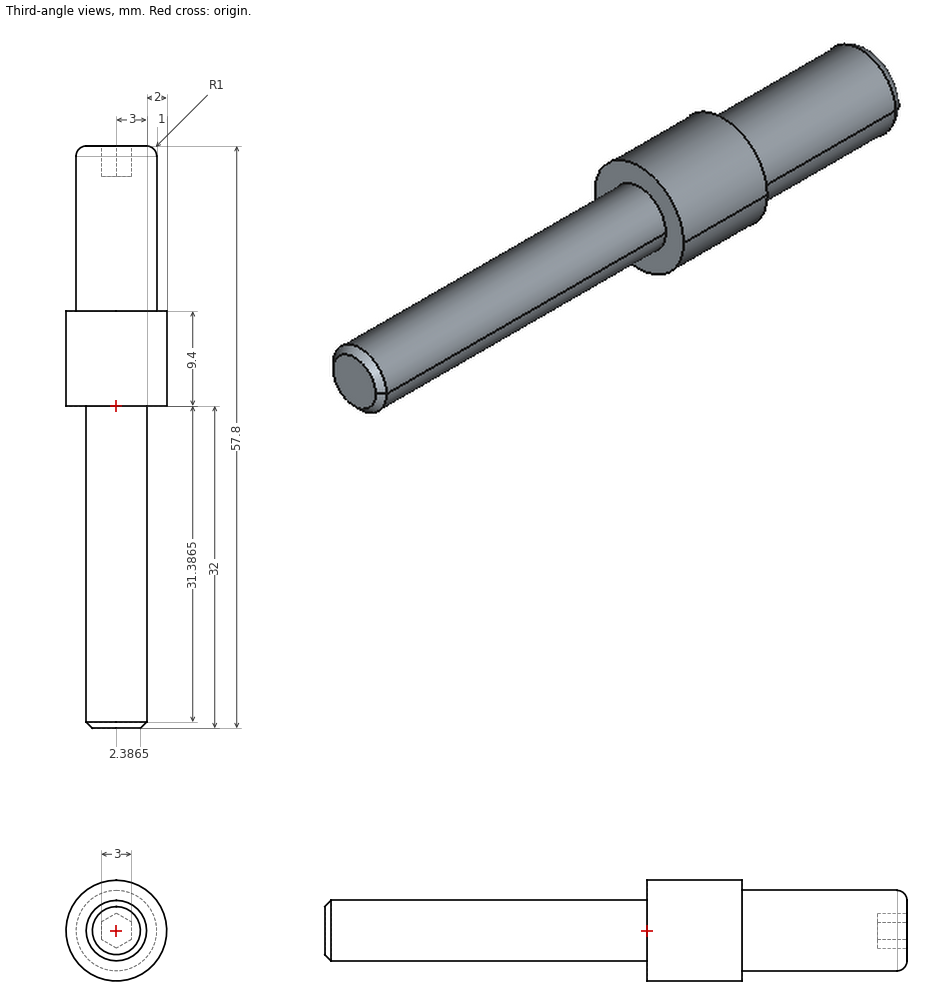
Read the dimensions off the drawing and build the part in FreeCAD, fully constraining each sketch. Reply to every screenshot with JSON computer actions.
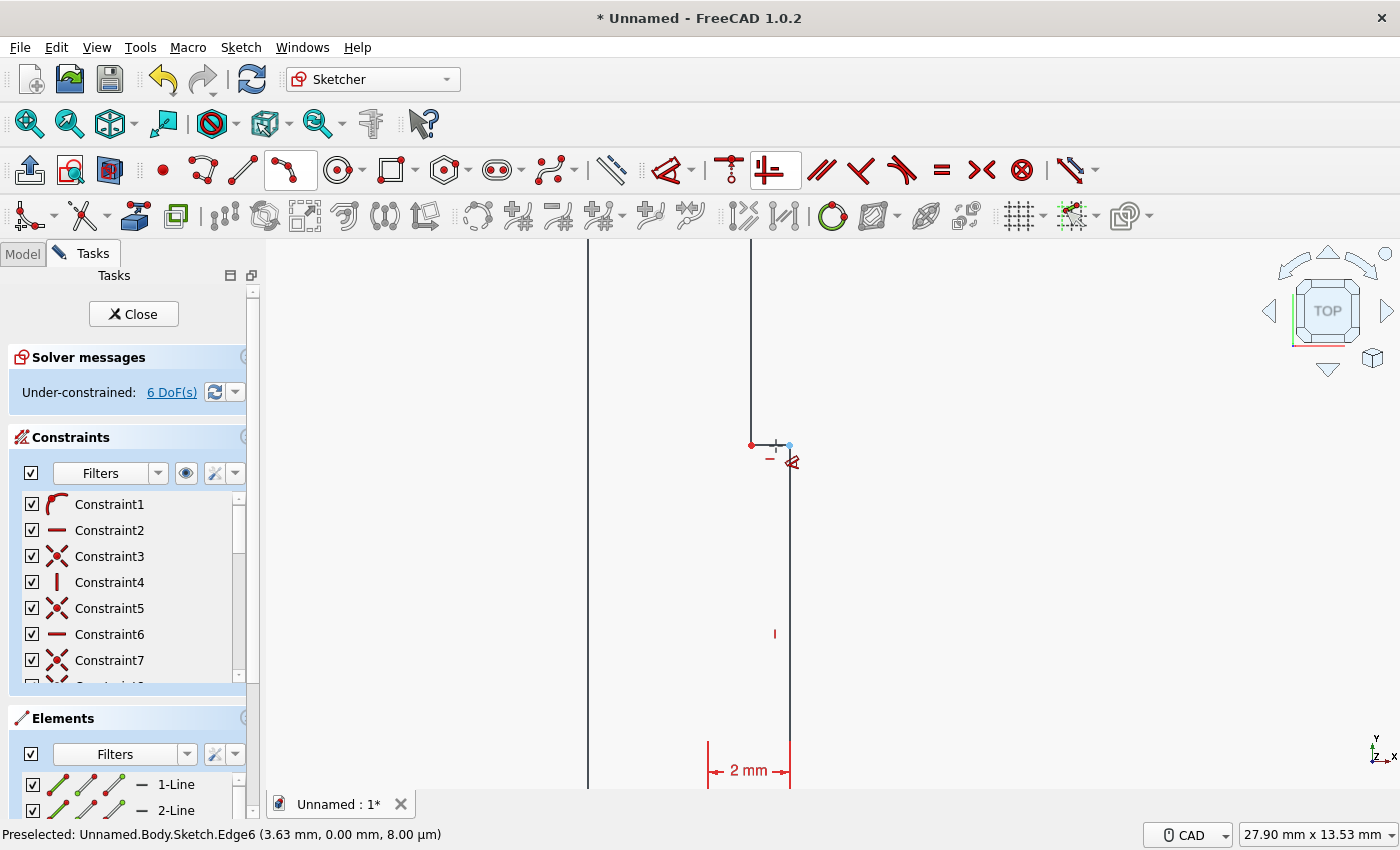
{"action": "left_click", "coordinate": [774, 445]}
{"action": "left_click", "coordinate": [770, 411]}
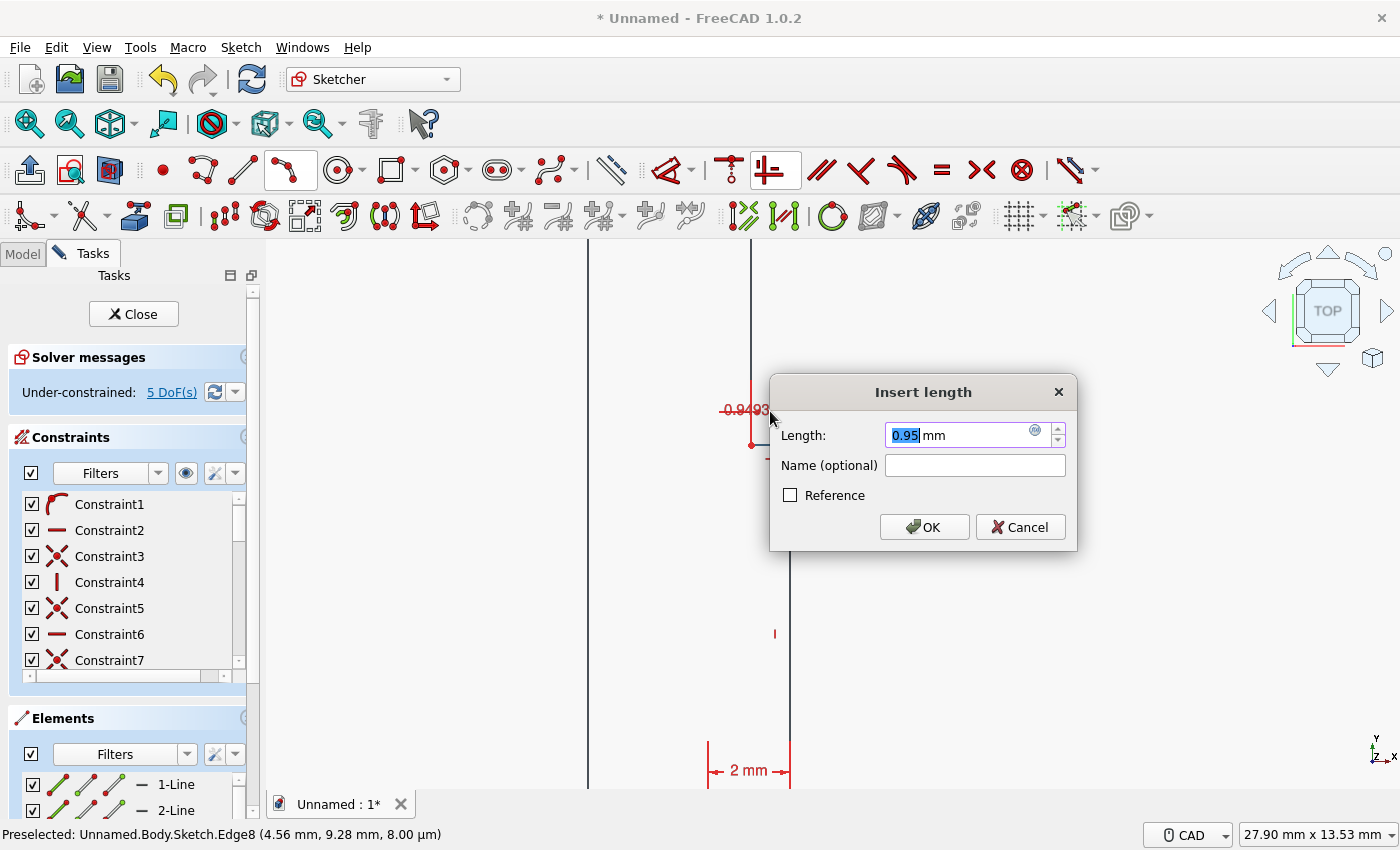
{"action": "type", "text": "1"}
{"action": "key", "text": "Return"}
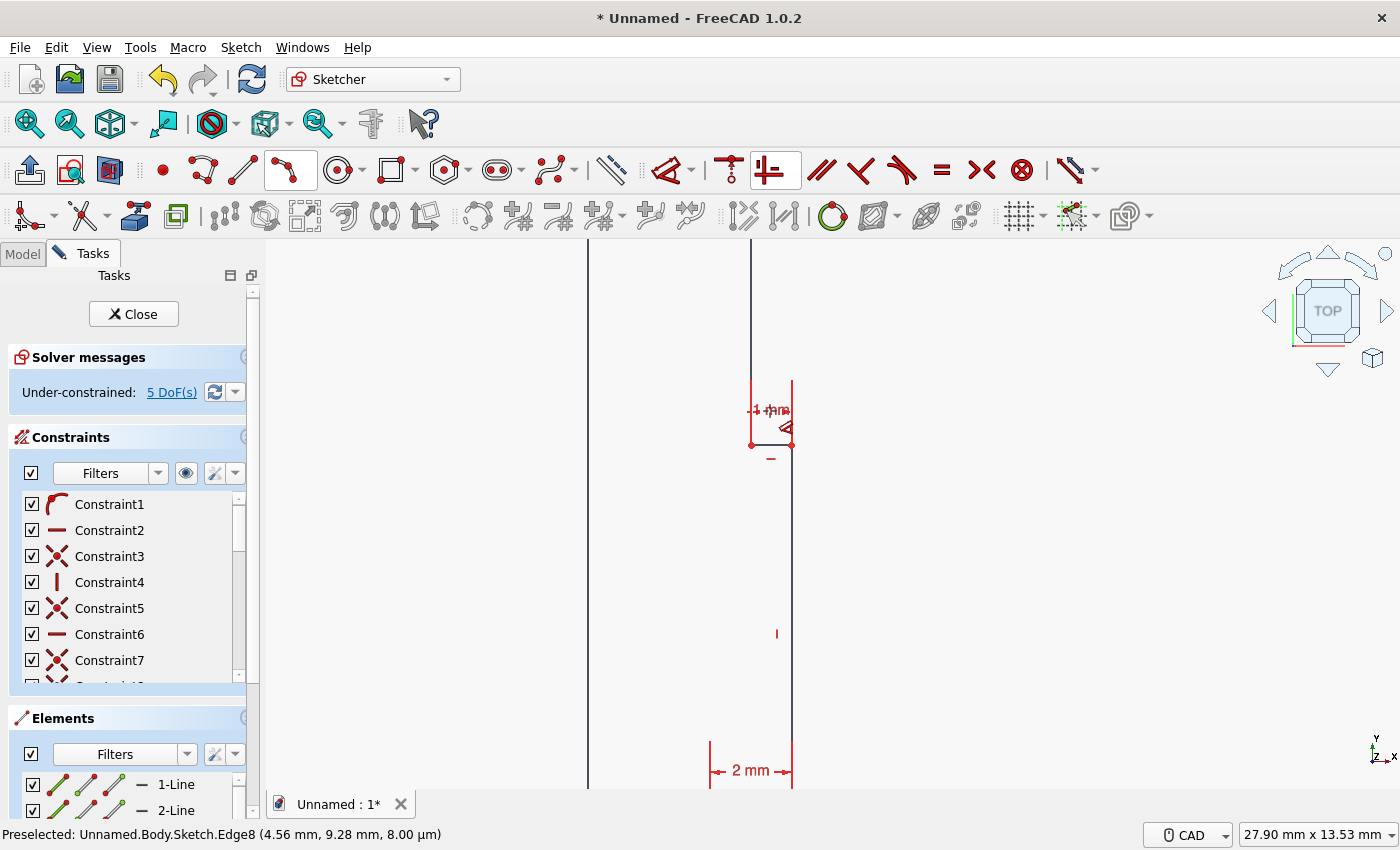
{"action": "scroll", "coordinate": [776, 446], "scroll_direction": "down", "scroll_amount": 10}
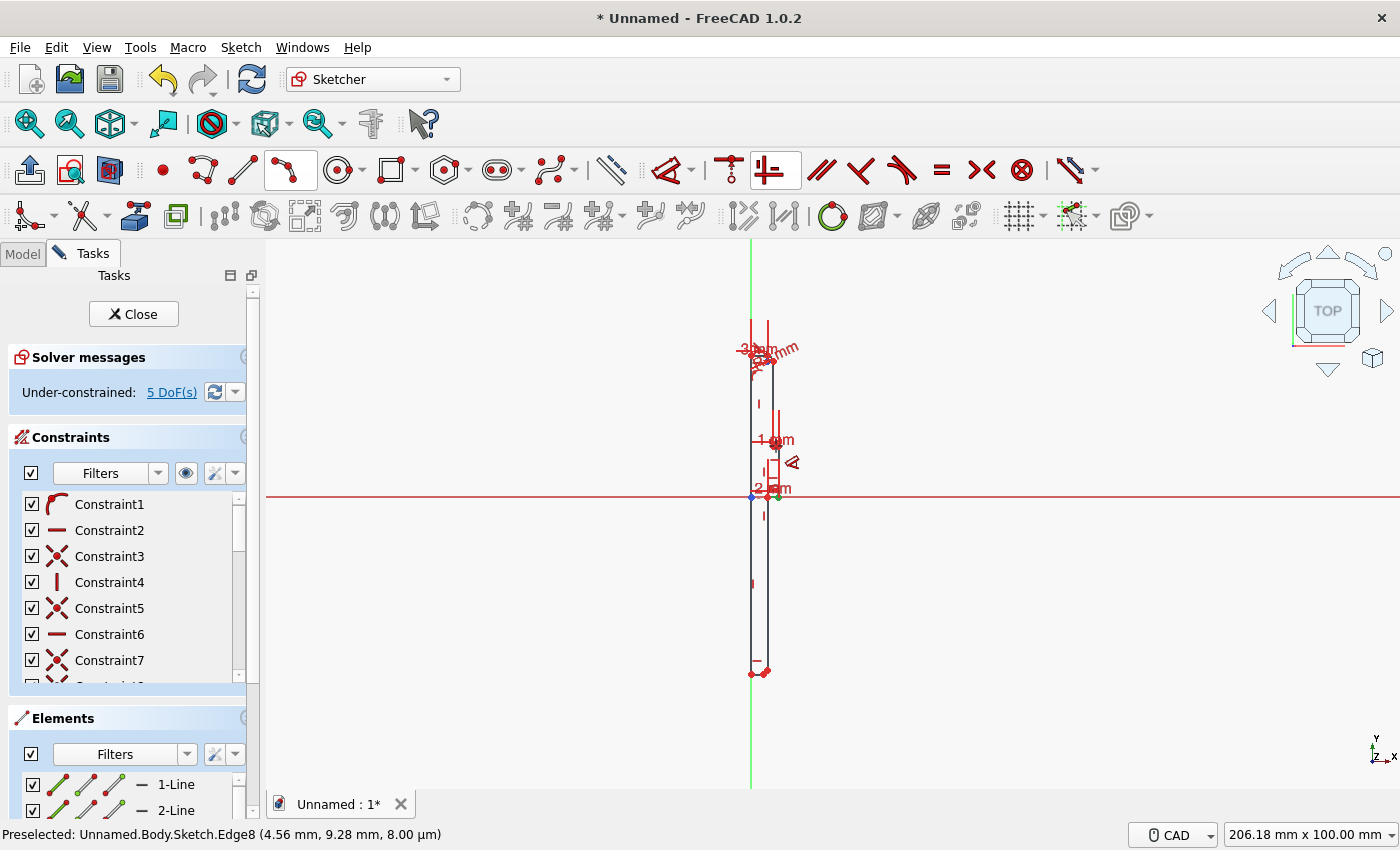
{"action": "left_click", "coordinate": [779, 482]}
{"action": "left_click", "coordinate": [861, 472]}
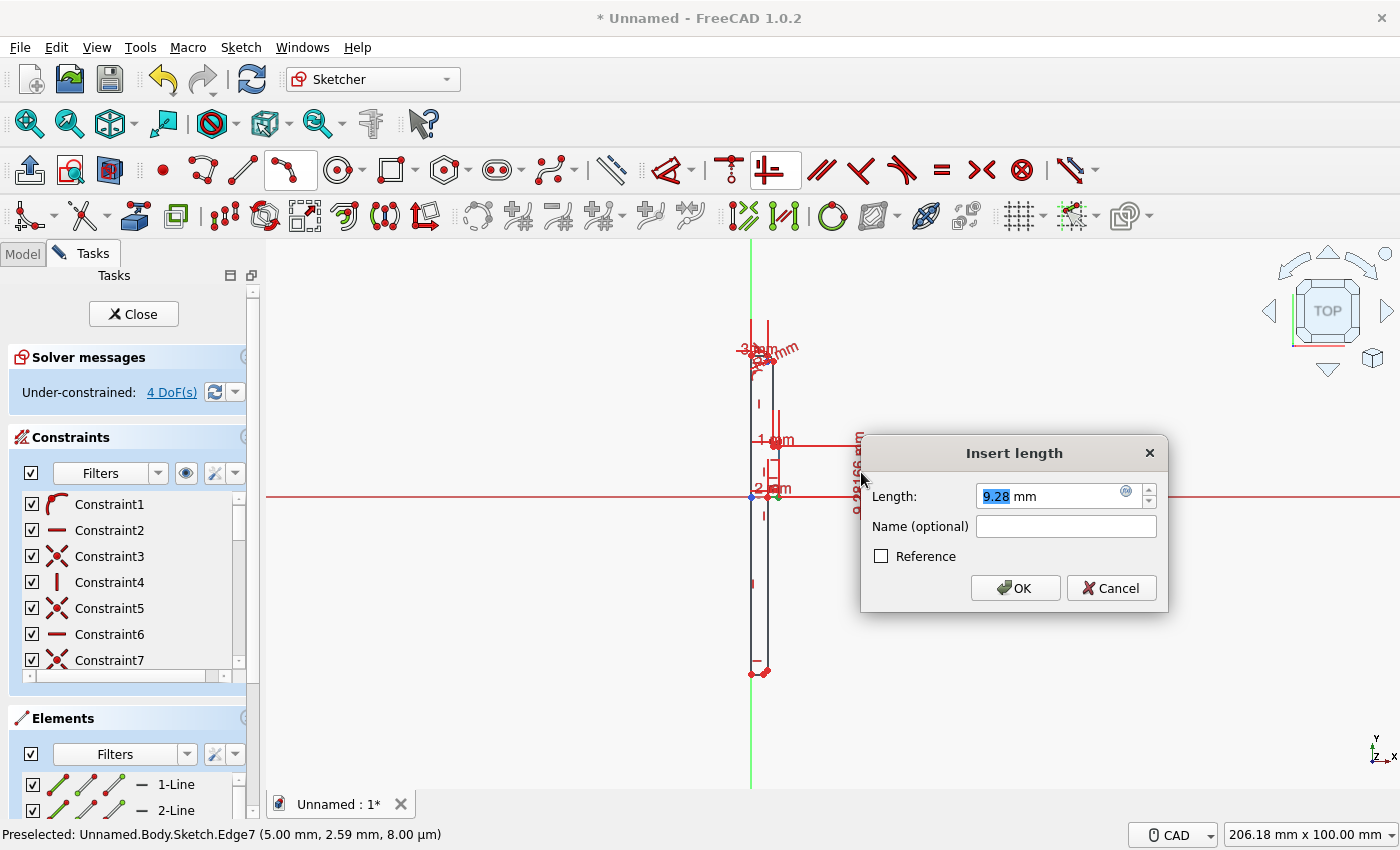
{"action": "type", "text": "9.4"}
{"action": "key", "text": "Return"}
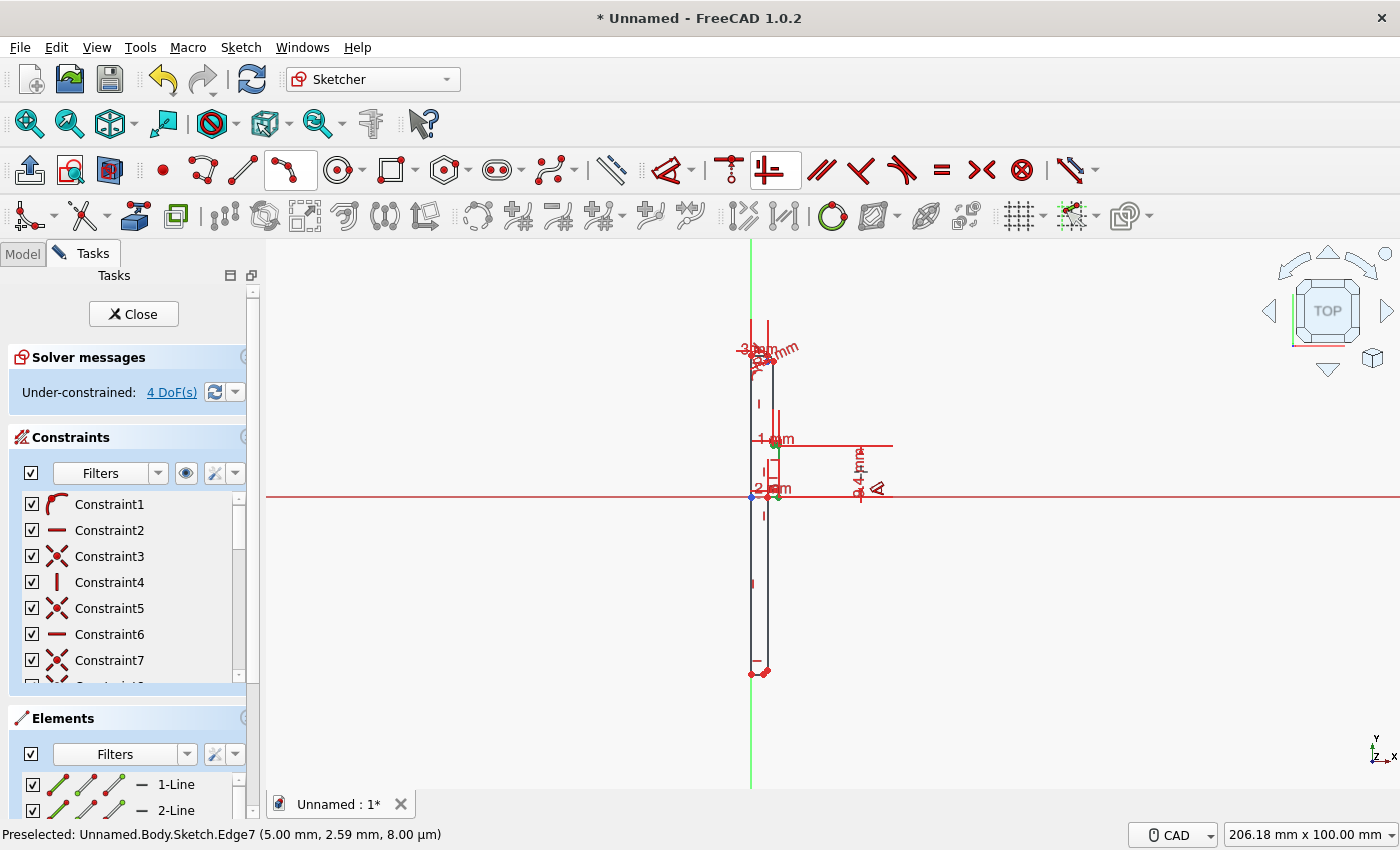
{"action": "left_click", "coordinate": [751, 675]}
{"action": "left_click", "coordinate": [717, 586]}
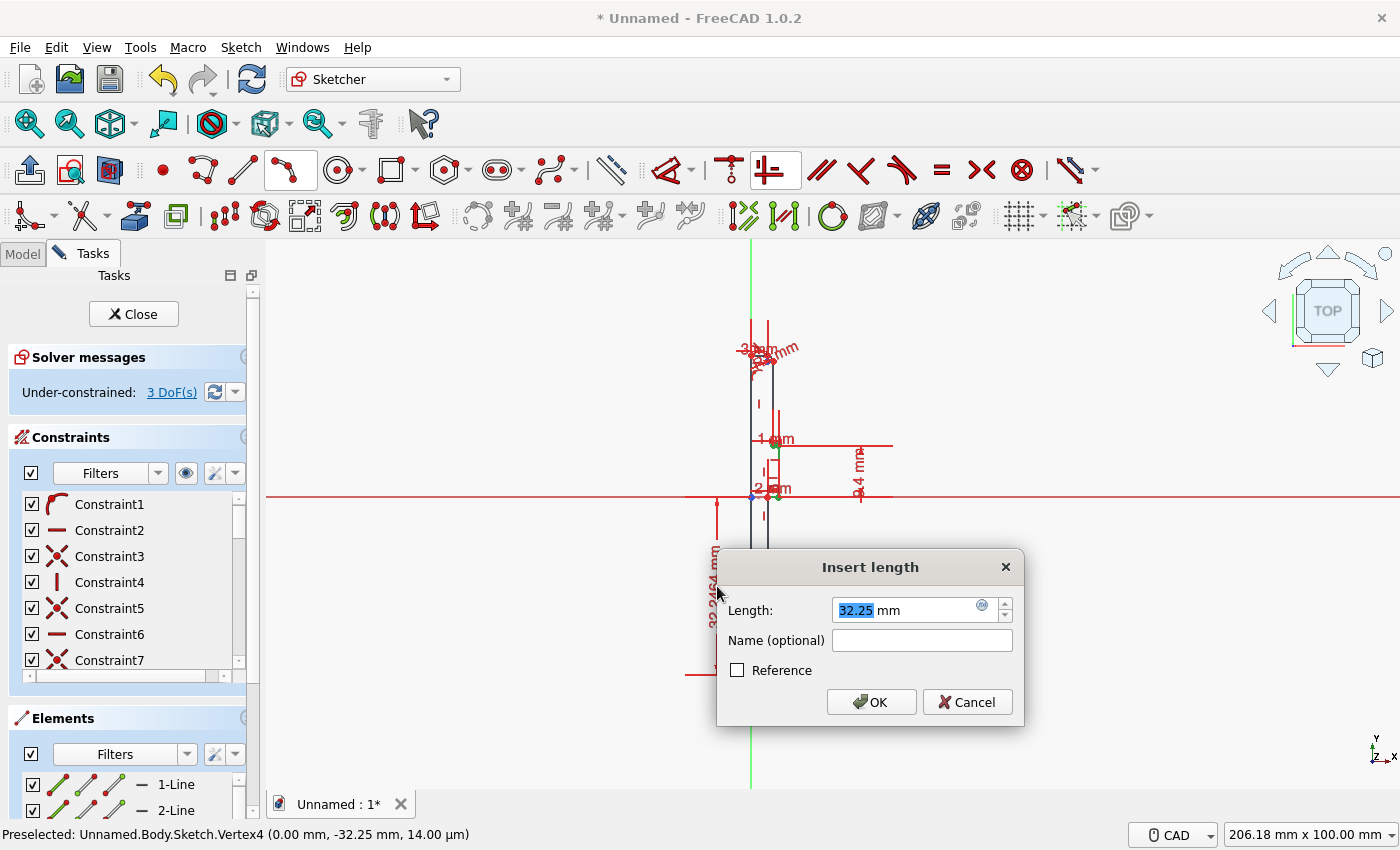
{"action": "type", "text": "32"}
{"action": "key", "text": "Return"}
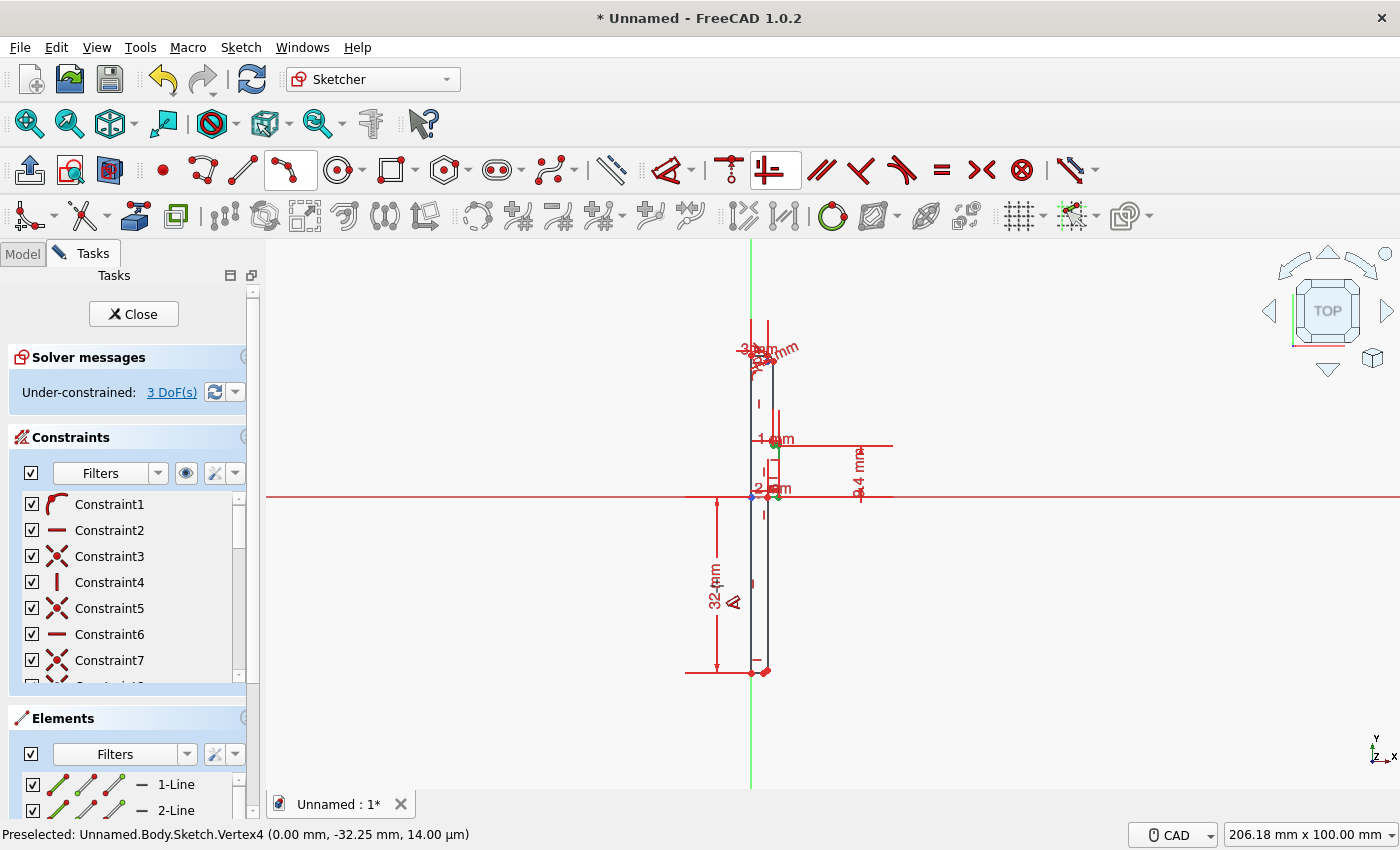
{"action": "left_click", "coordinate": [751, 451]}
{"action": "left_click", "coordinate": [717, 515]}